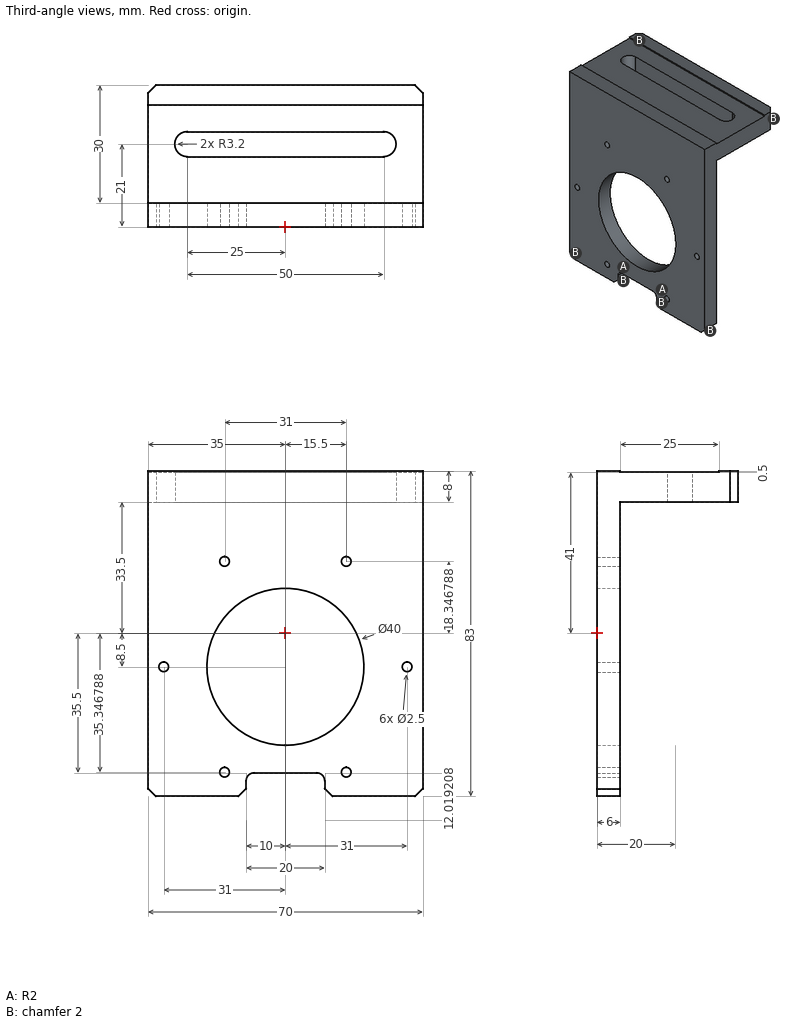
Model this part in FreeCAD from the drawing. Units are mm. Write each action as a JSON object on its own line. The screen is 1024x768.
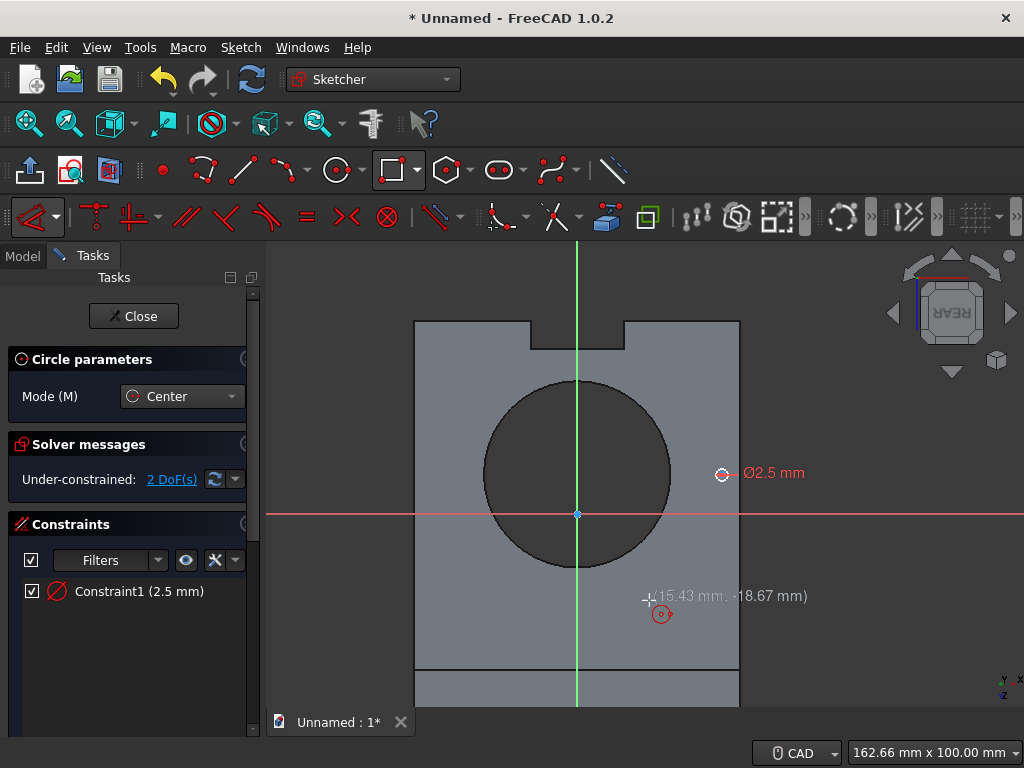
{"action": "left_click", "coordinate": [649, 600]}
{"action": "mouse_move", "coordinate": [653, 595]}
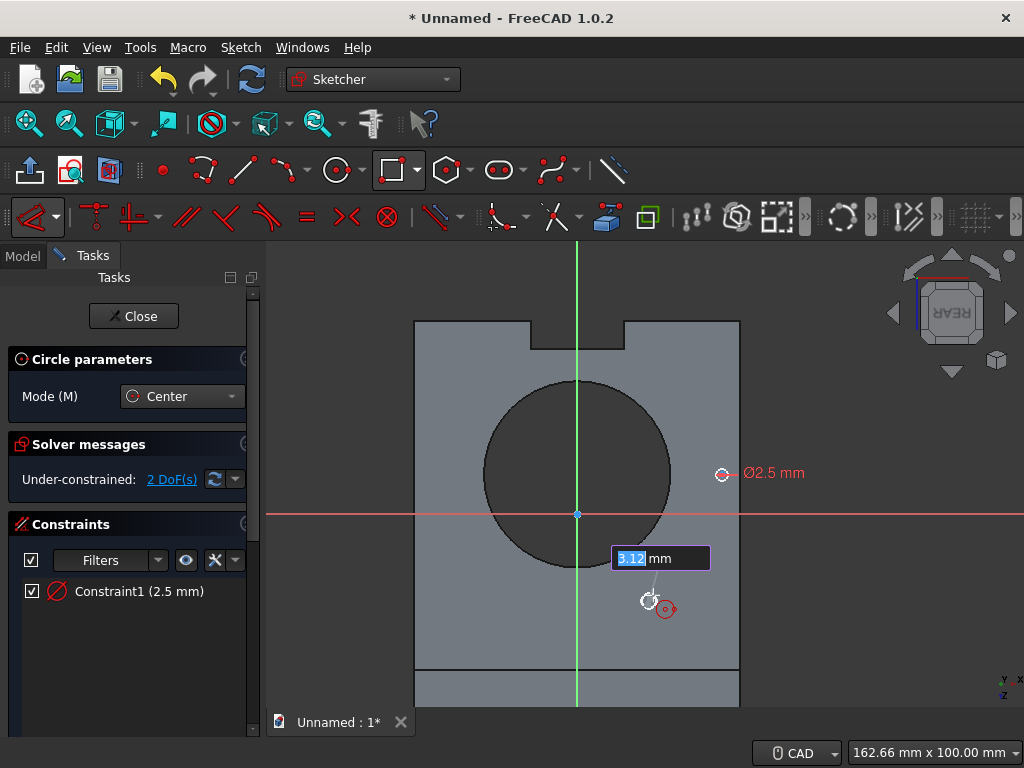
{"action": "type", "text": "2.5"}
{"action": "key", "text": "Return"}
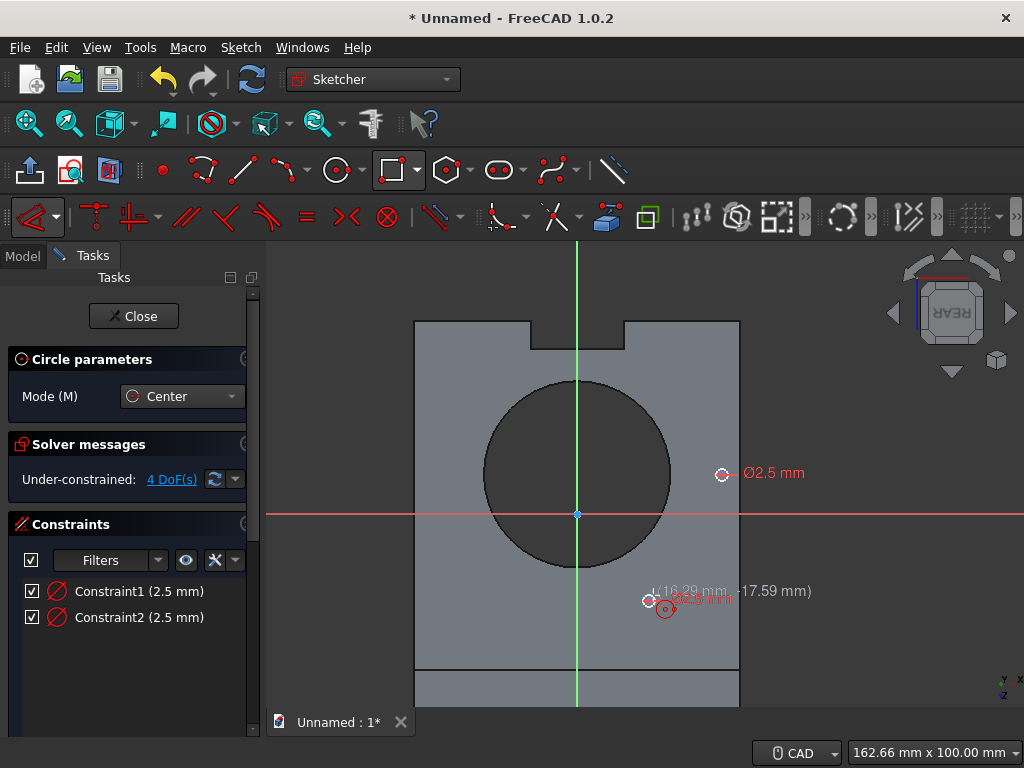
{"action": "scroll", "coordinate": [505, 600], "scroll_direction": "up", "scroll_amount": 7}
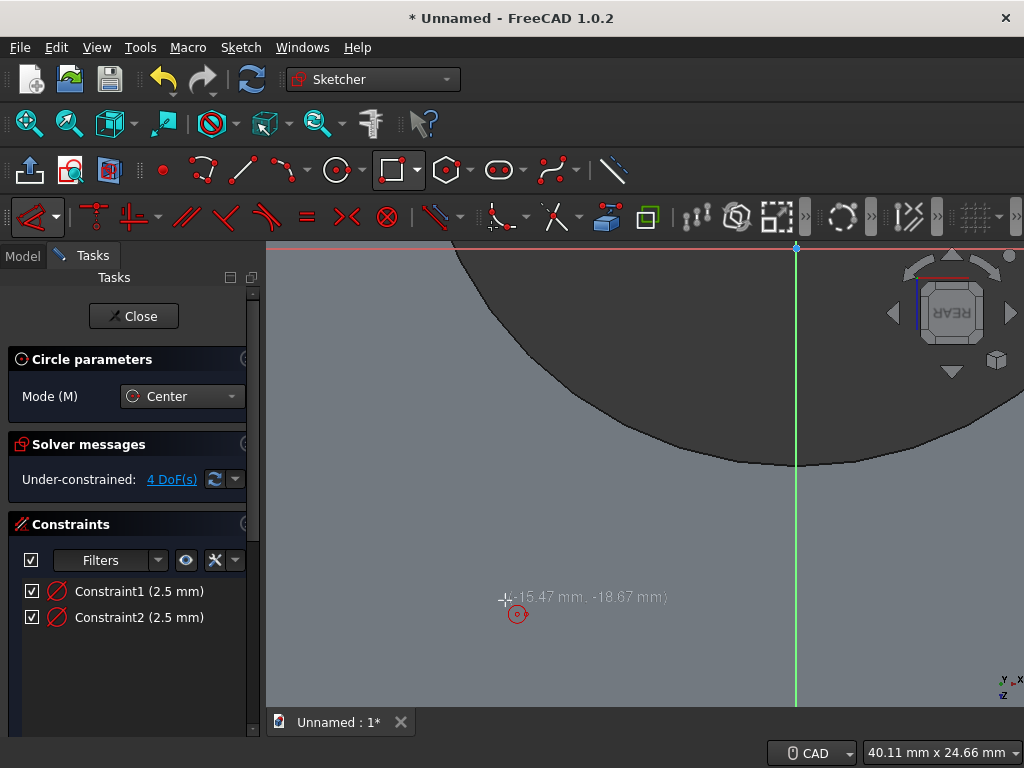
{"action": "scroll", "coordinate": [505, 600], "scroll_direction": "down", "scroll_amount": 7}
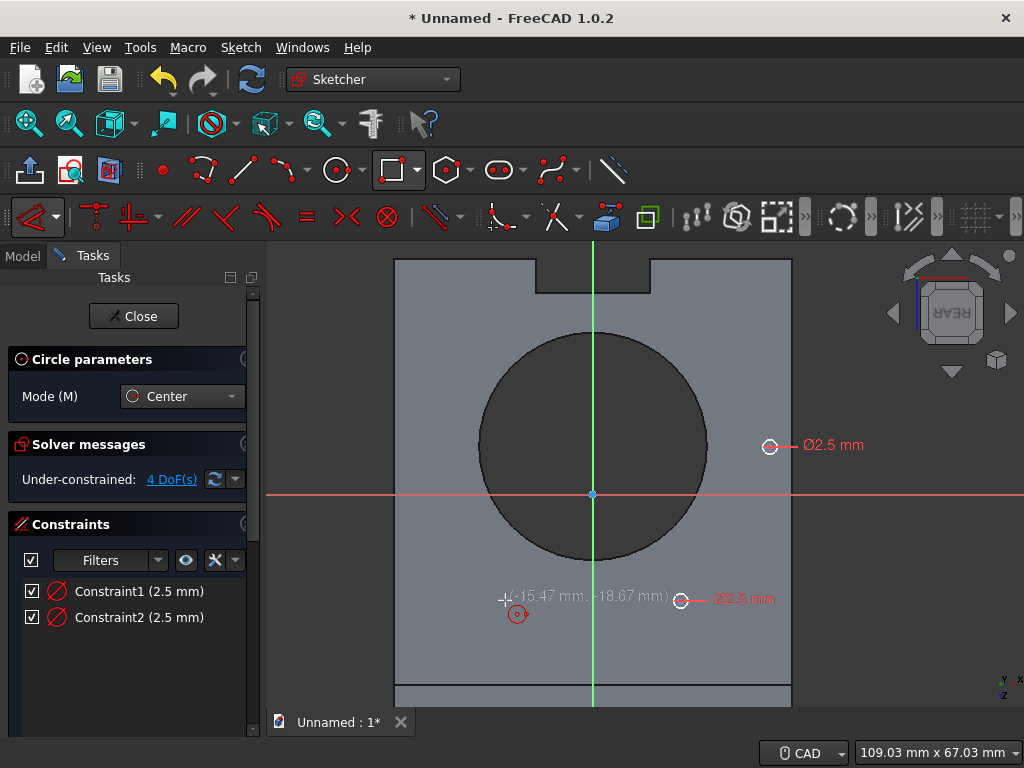
{"action": "left_click", "coordinate": [505, 600]}
{"action": "mouse_move", "coordinate": [509, 595]}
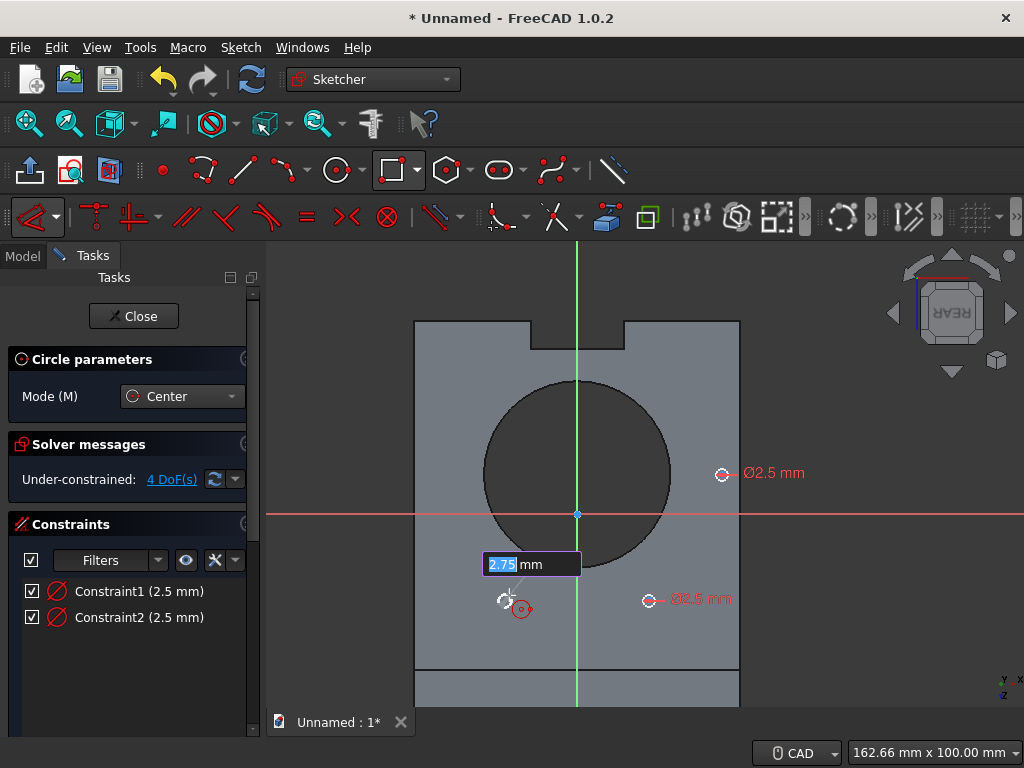
{"action": "type", "text": "2.5"}
{"action": "key", "text": "Return"}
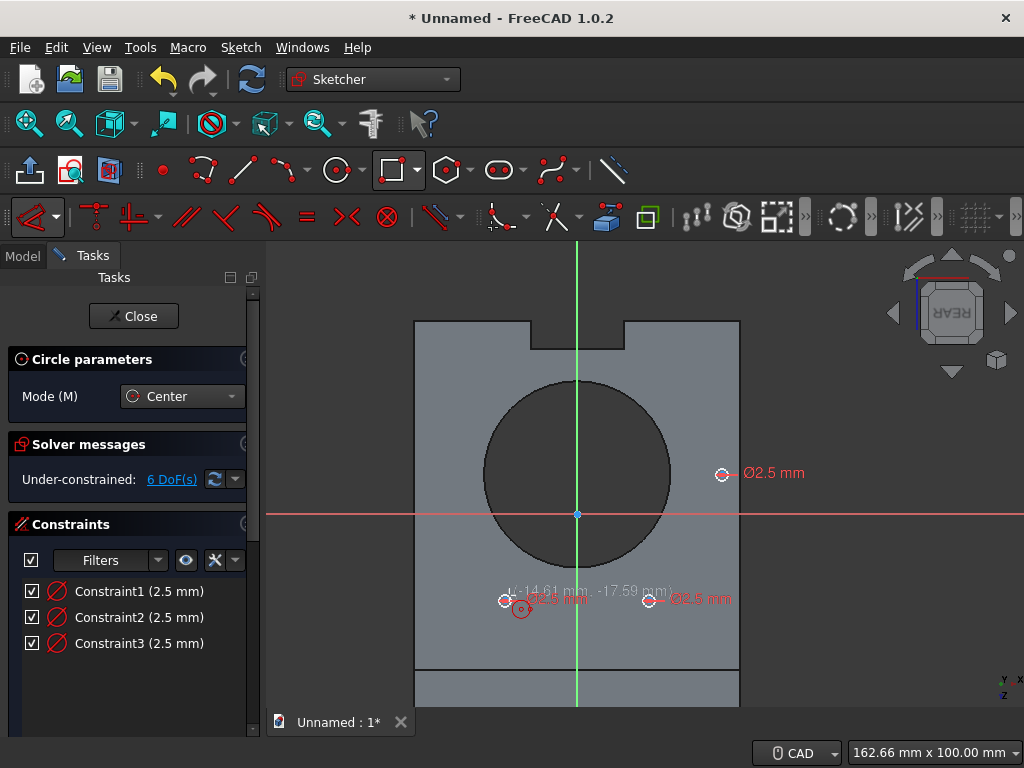
{"action": "scroll", "coordinate": [433, 474], "scroll_direction": "up", "scroll_amount": 7}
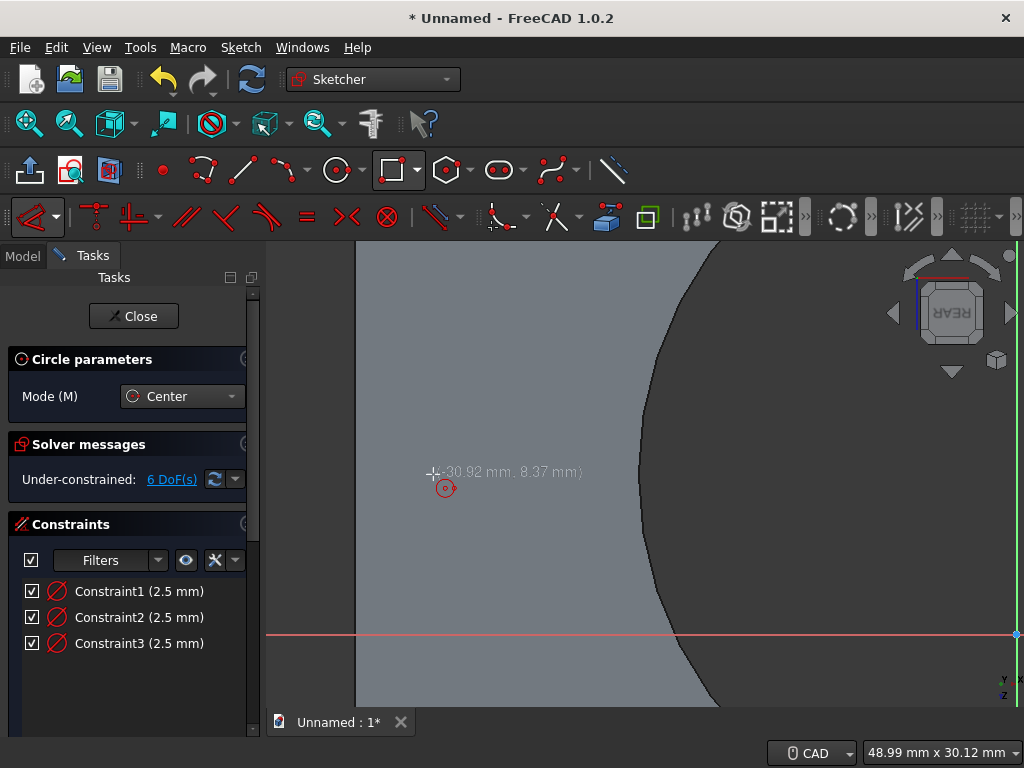
{"action": "scroll", "coordinate": [432, 474], "scroll_direction": "down", "scroll_amount": 7}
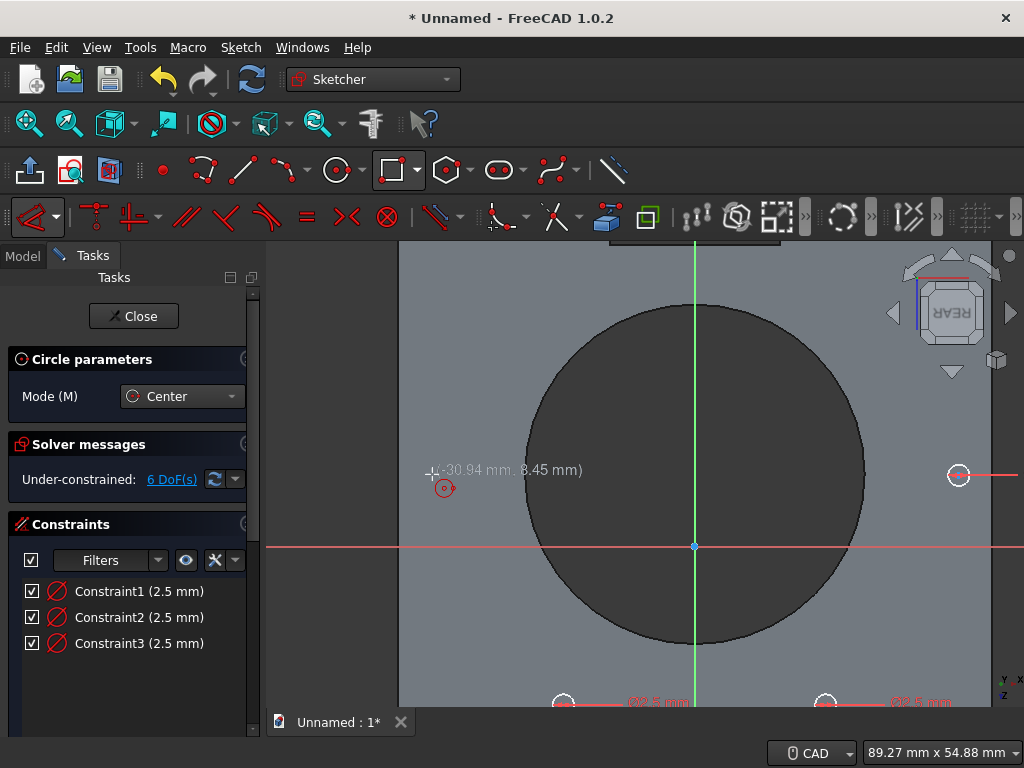
{"action": "left_click", "coordinate": [432, 474]}
{"action": "mouse_move", "coordinate": [436, 470]}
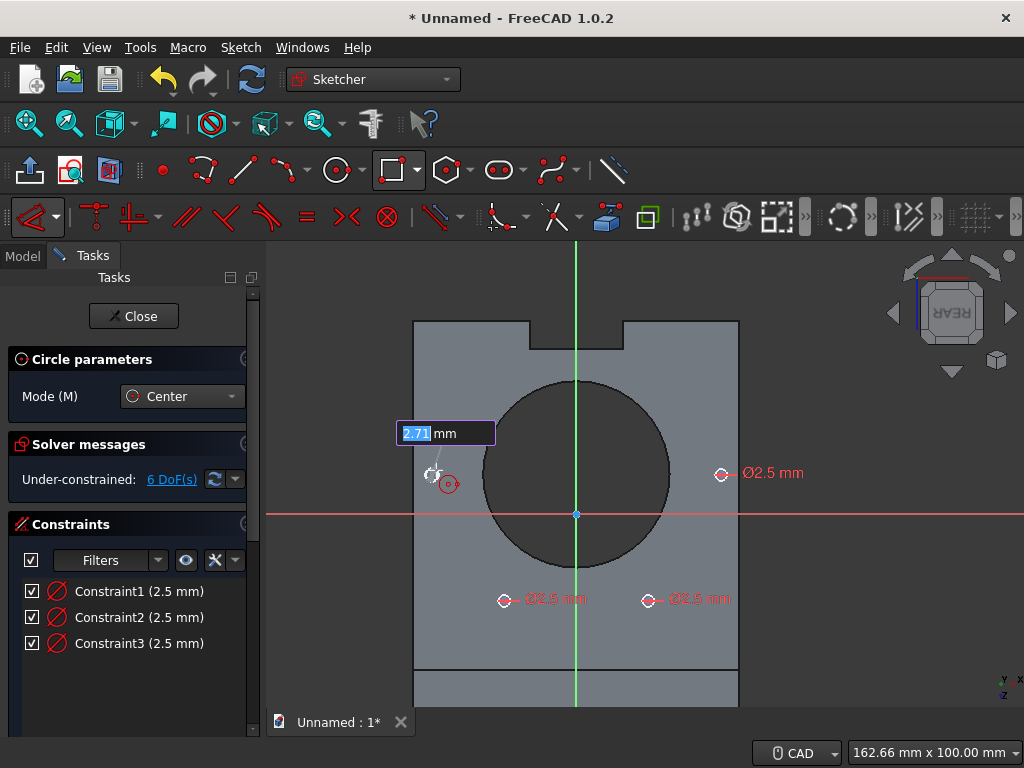
{"action": "type", "text": "2.5"}
{"action": "key", "text": "Return"}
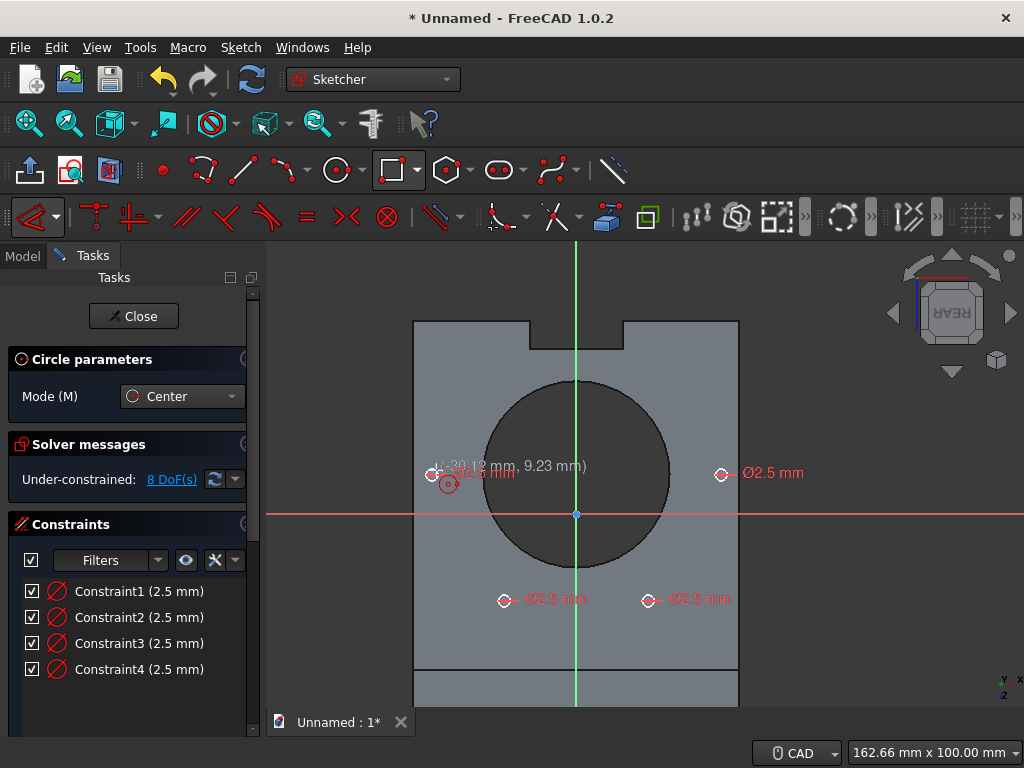
{"action": "scroll", "coordinate": [504, 349], "scroll_direction": "up", "scroll_amount": 7}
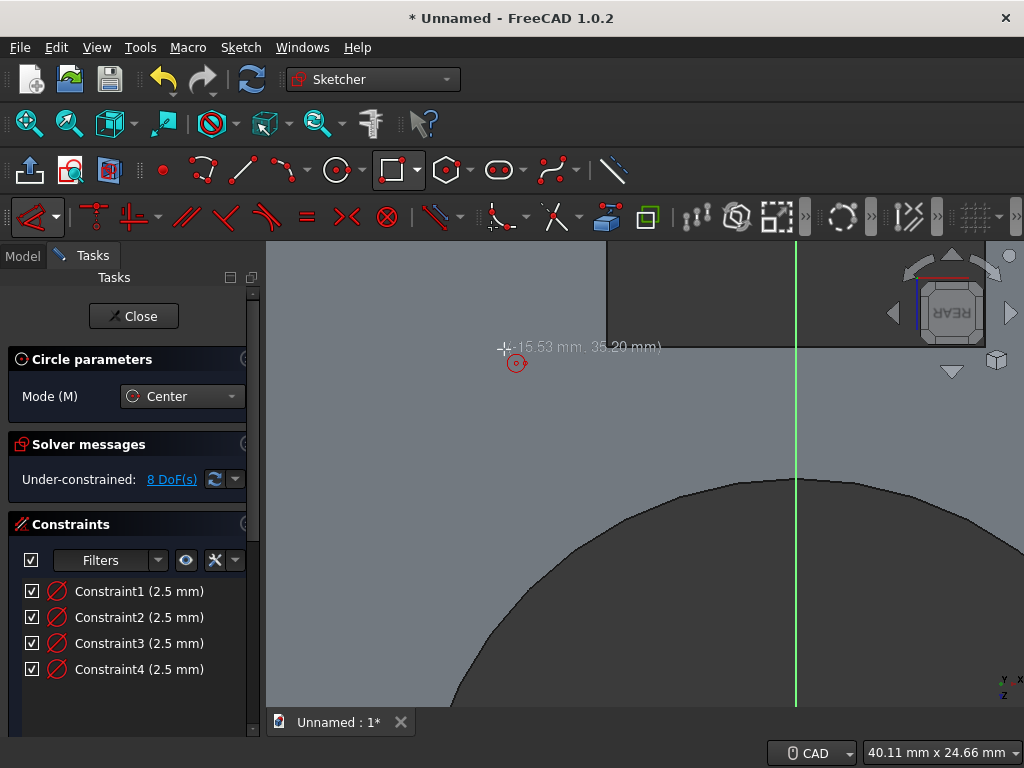
{"action": "scroll", "coordinate": [505, 349], "scroll_direction": "down", "scroll_amount": 7}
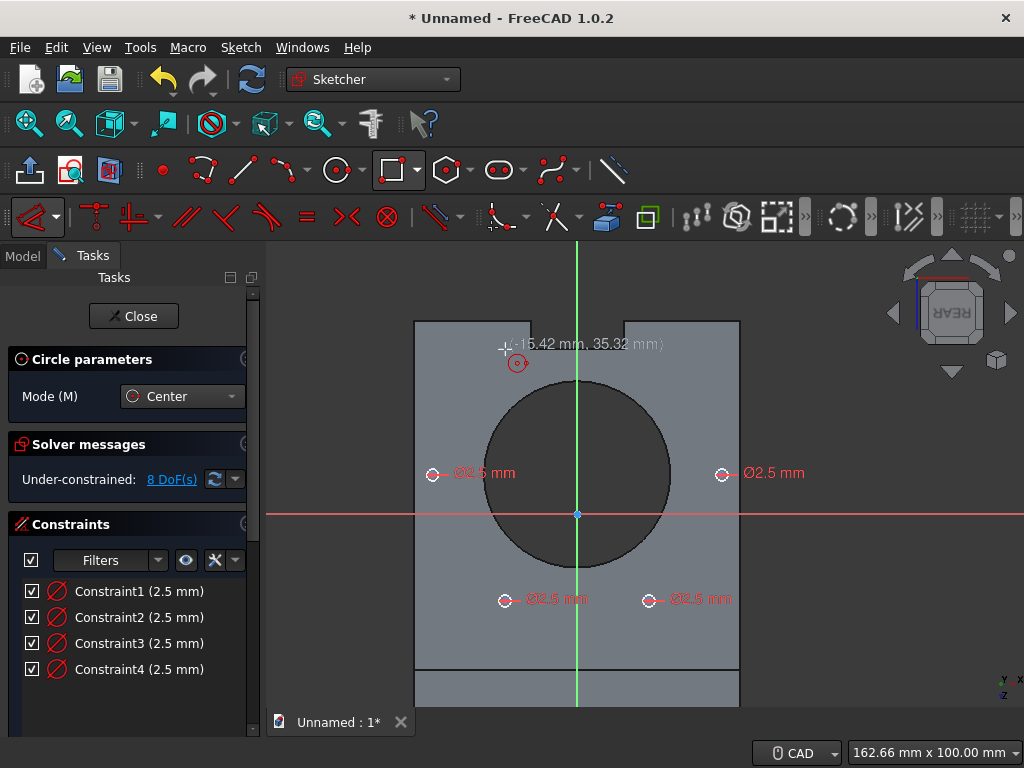
{"action": "left_click", "coordinate": [505, 349]}
{"action": "mouse_move", "coordinate": [509, 345]}